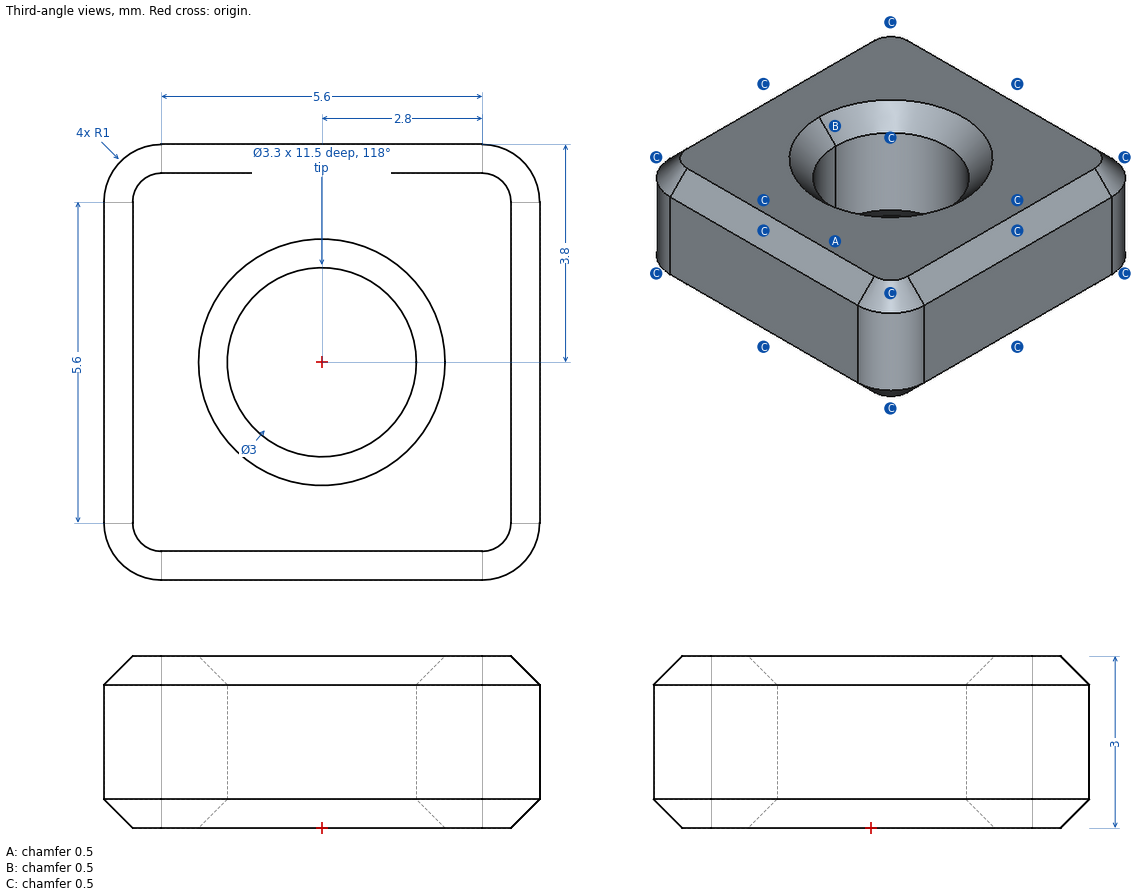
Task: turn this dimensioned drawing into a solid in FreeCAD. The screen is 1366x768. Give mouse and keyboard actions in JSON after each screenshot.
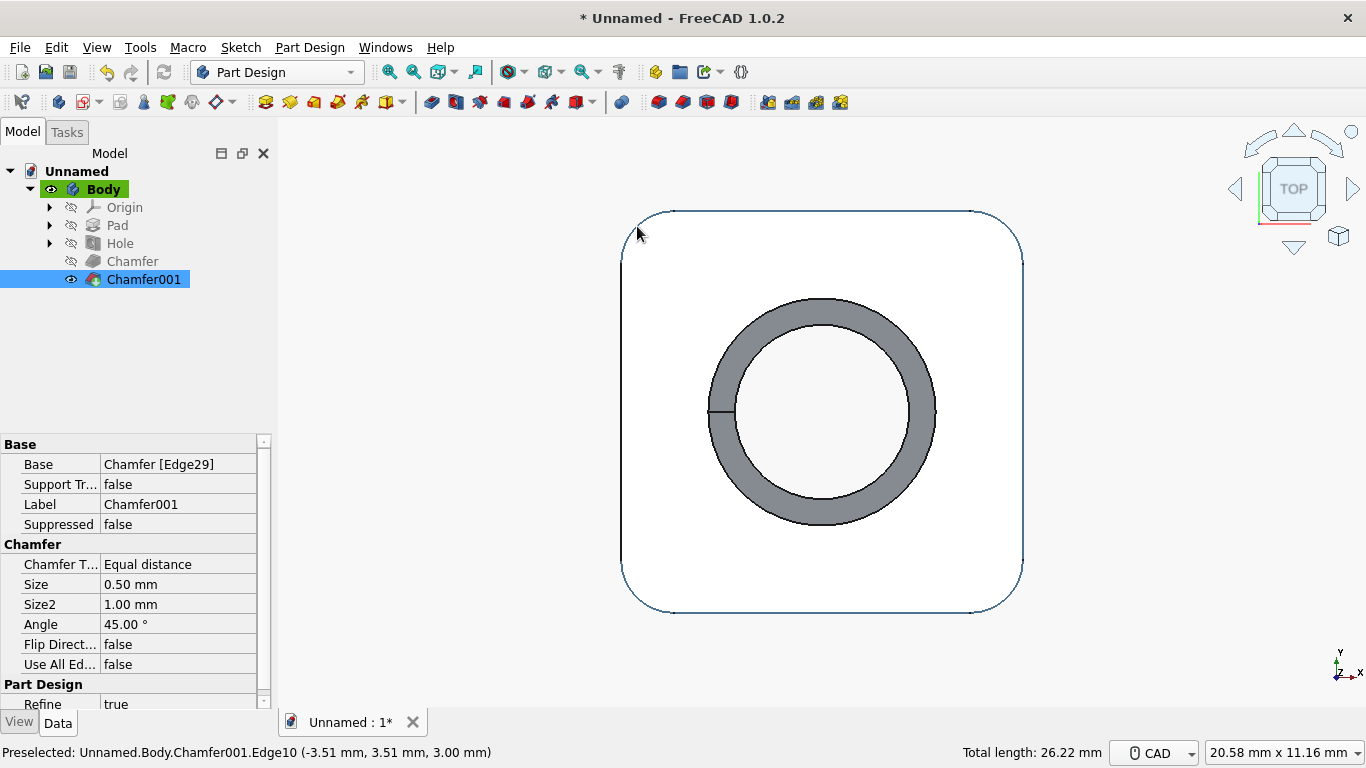
{"action": "left_click", "coordinate": [621, 411], "text": "ctrl"}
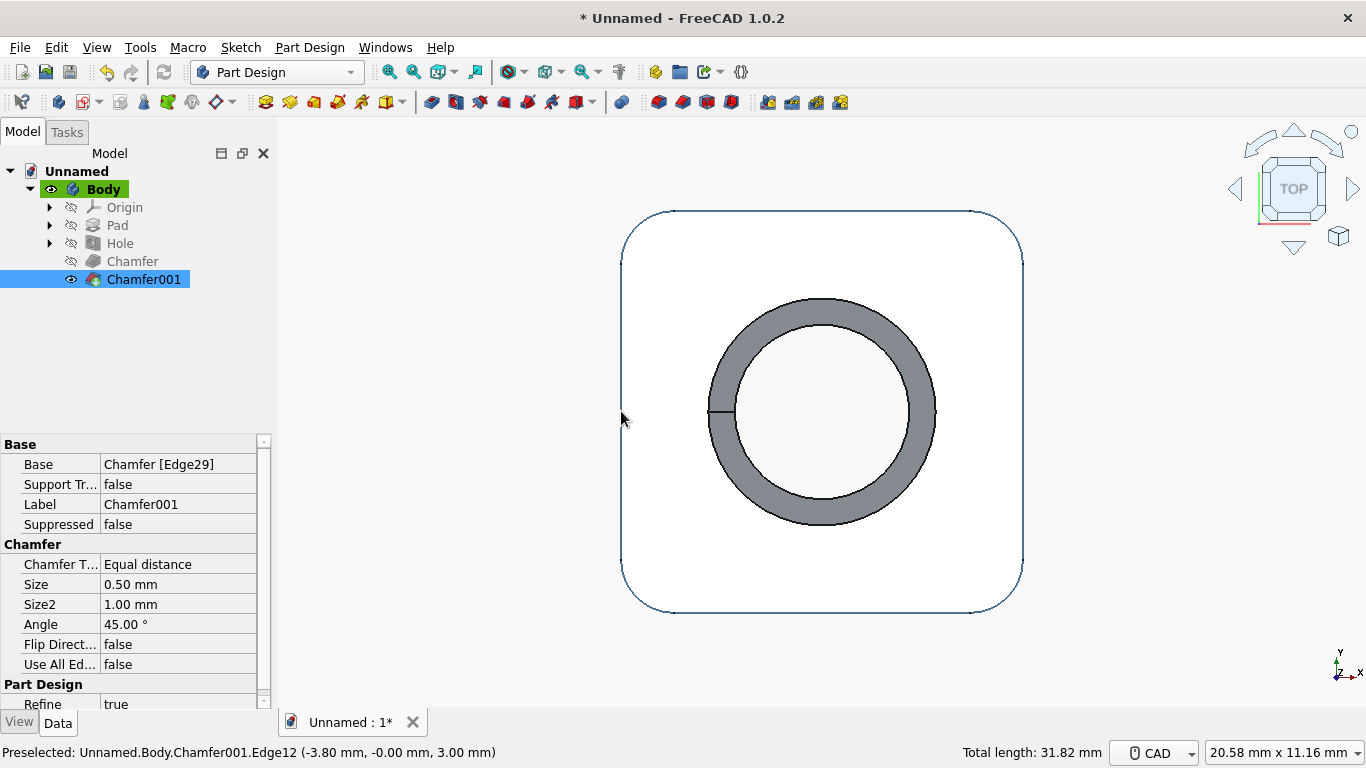
{"action": "key", "text": "0"}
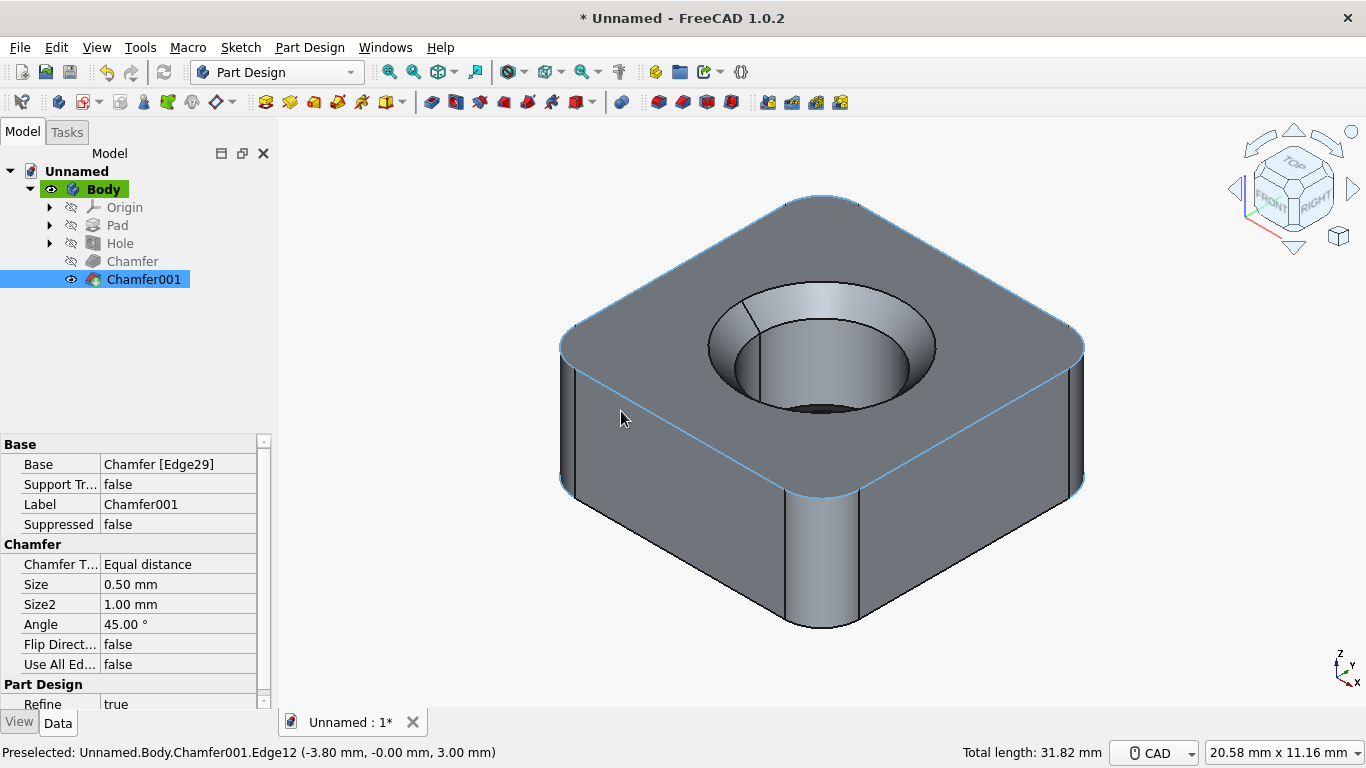
{"action": "key", "text": "1"}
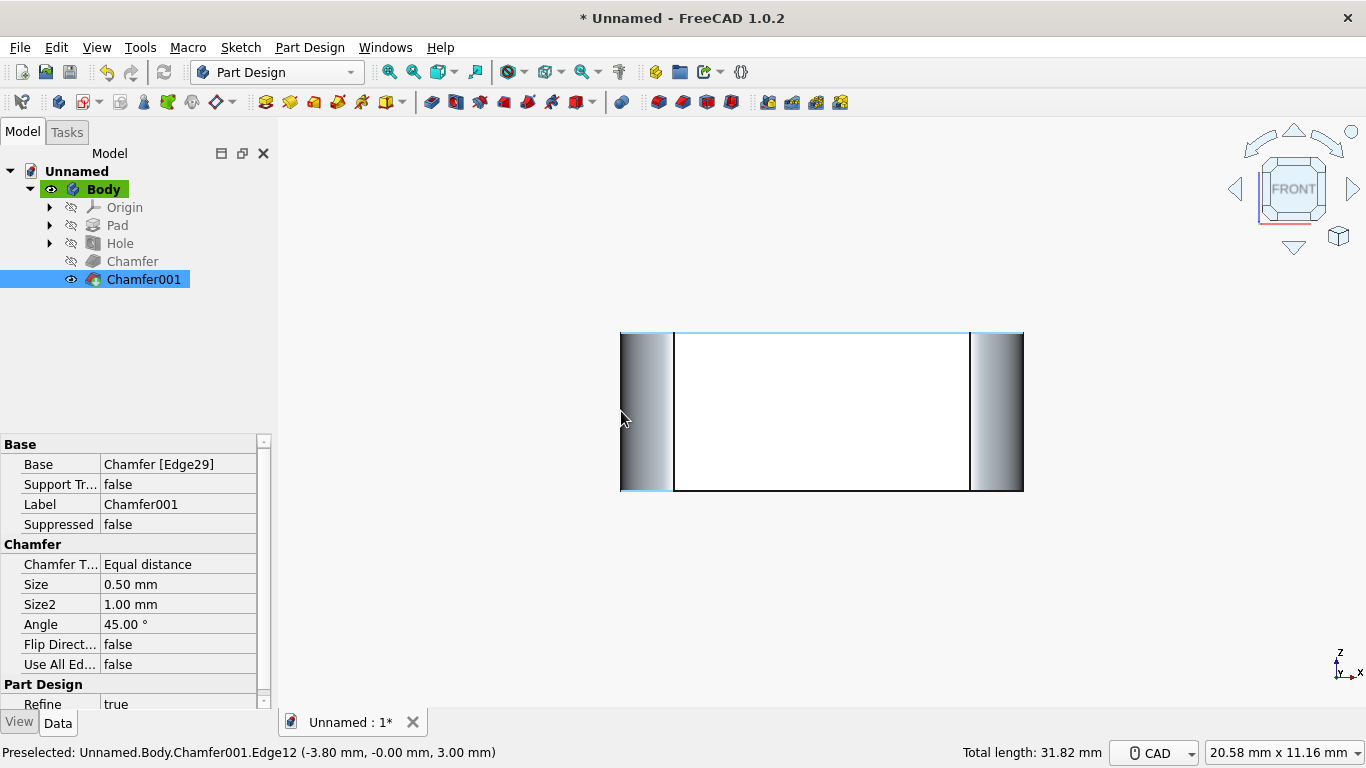
{"action": "key", "text": "v f"}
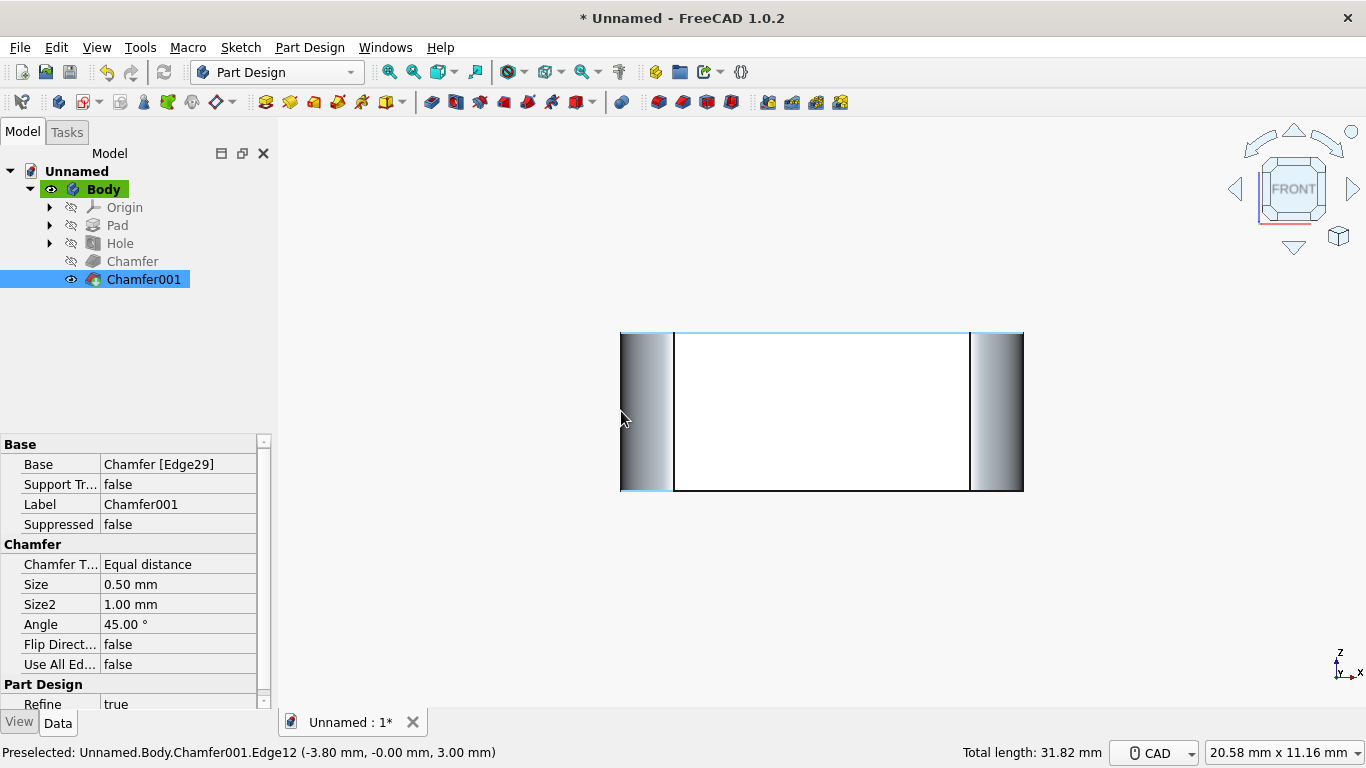
{"action": "left_click", "coordinate": [822, 490], "text": "ctrl"}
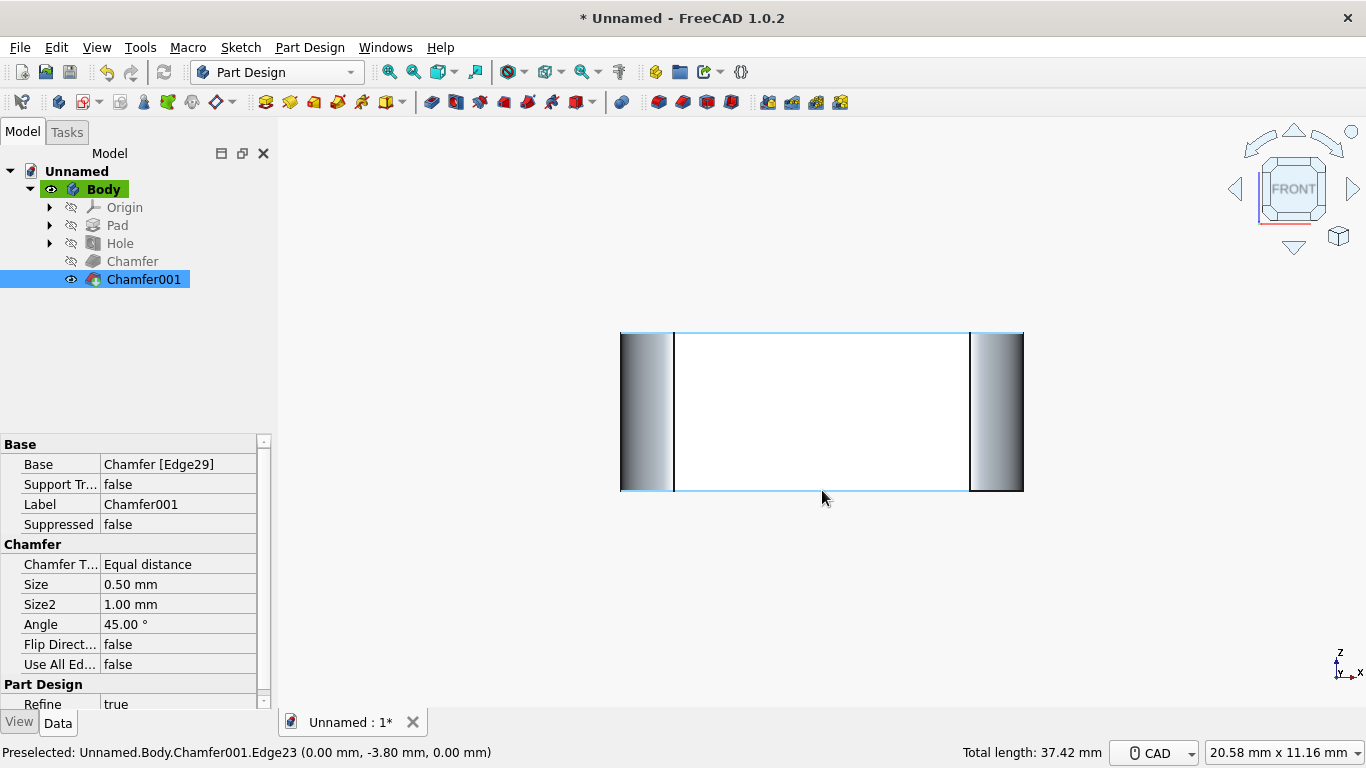
{"action": "left_click", "coordinate": [1007, 490], "text": "ctrl"}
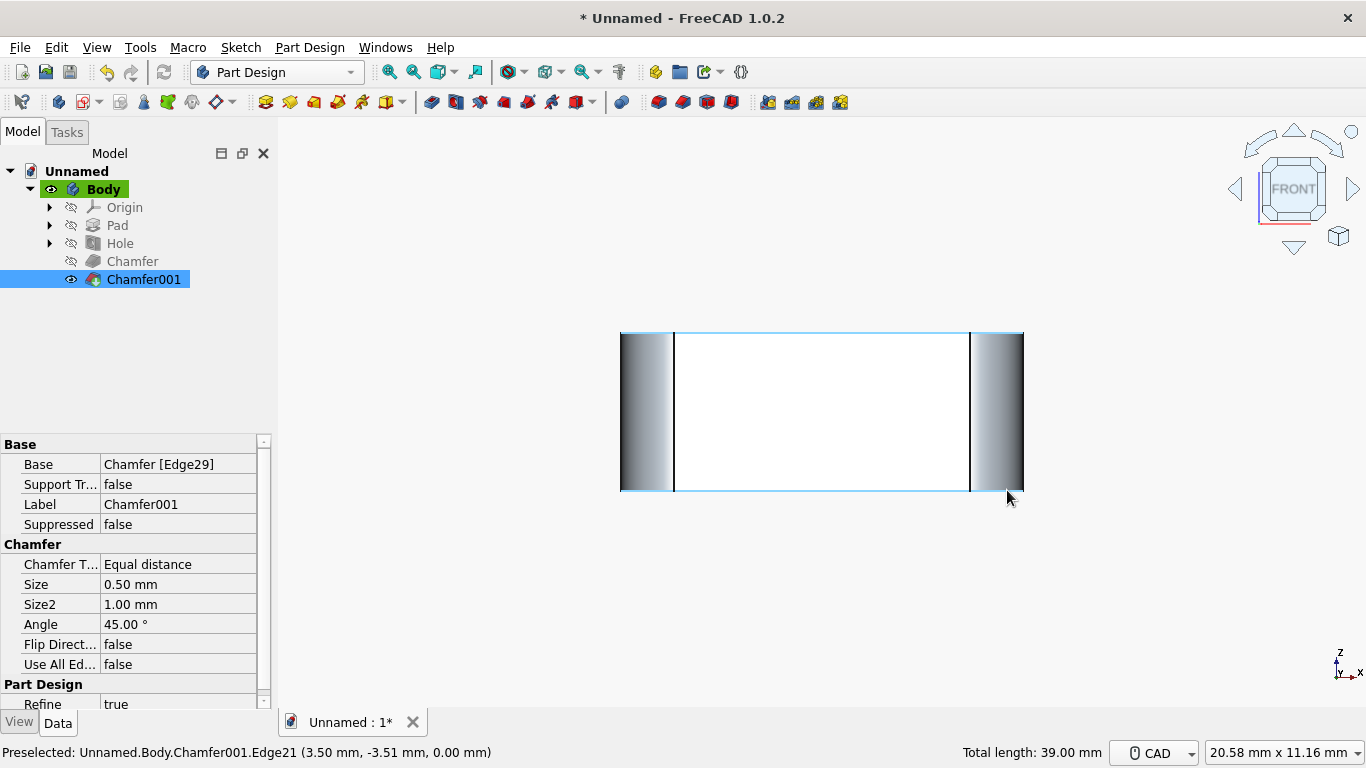
{"action": "key", "text": "3"}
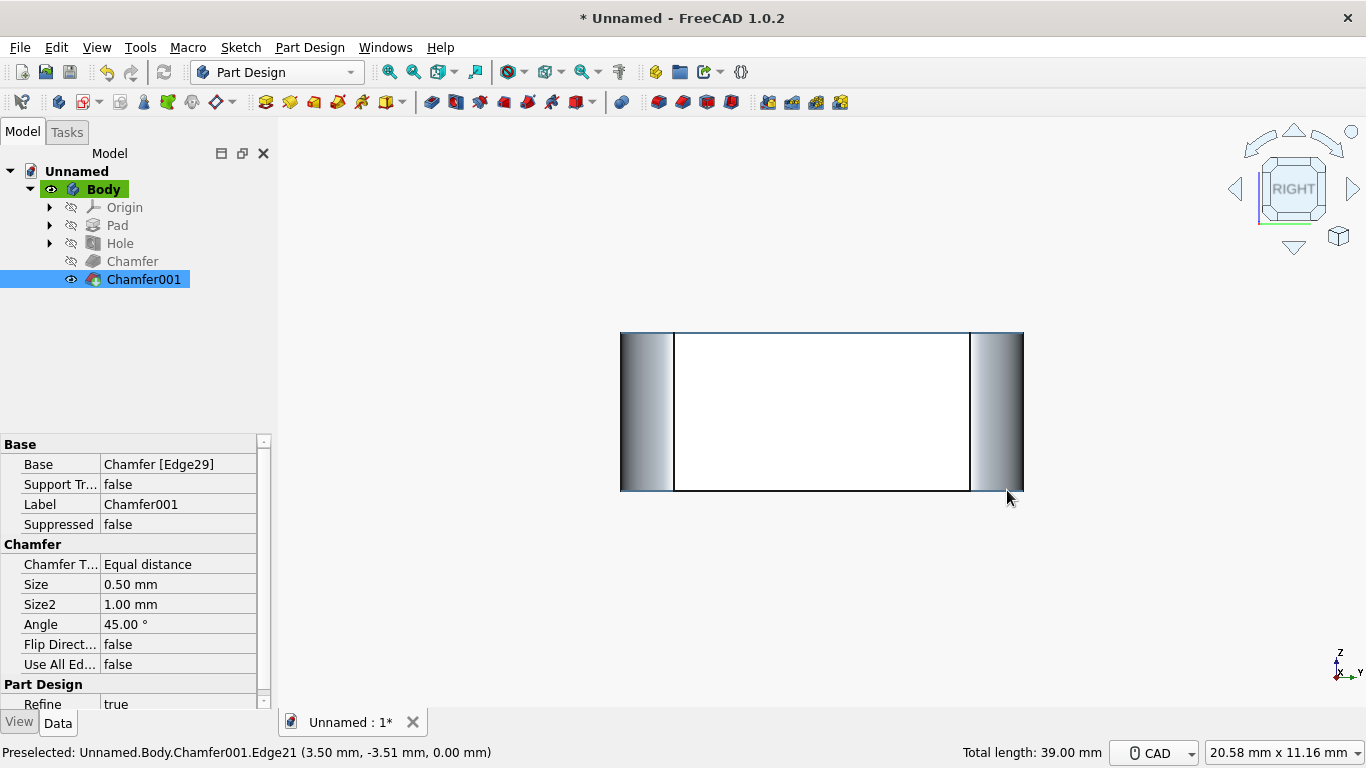
{"action": "left_click", "coordinate": [390, 72]}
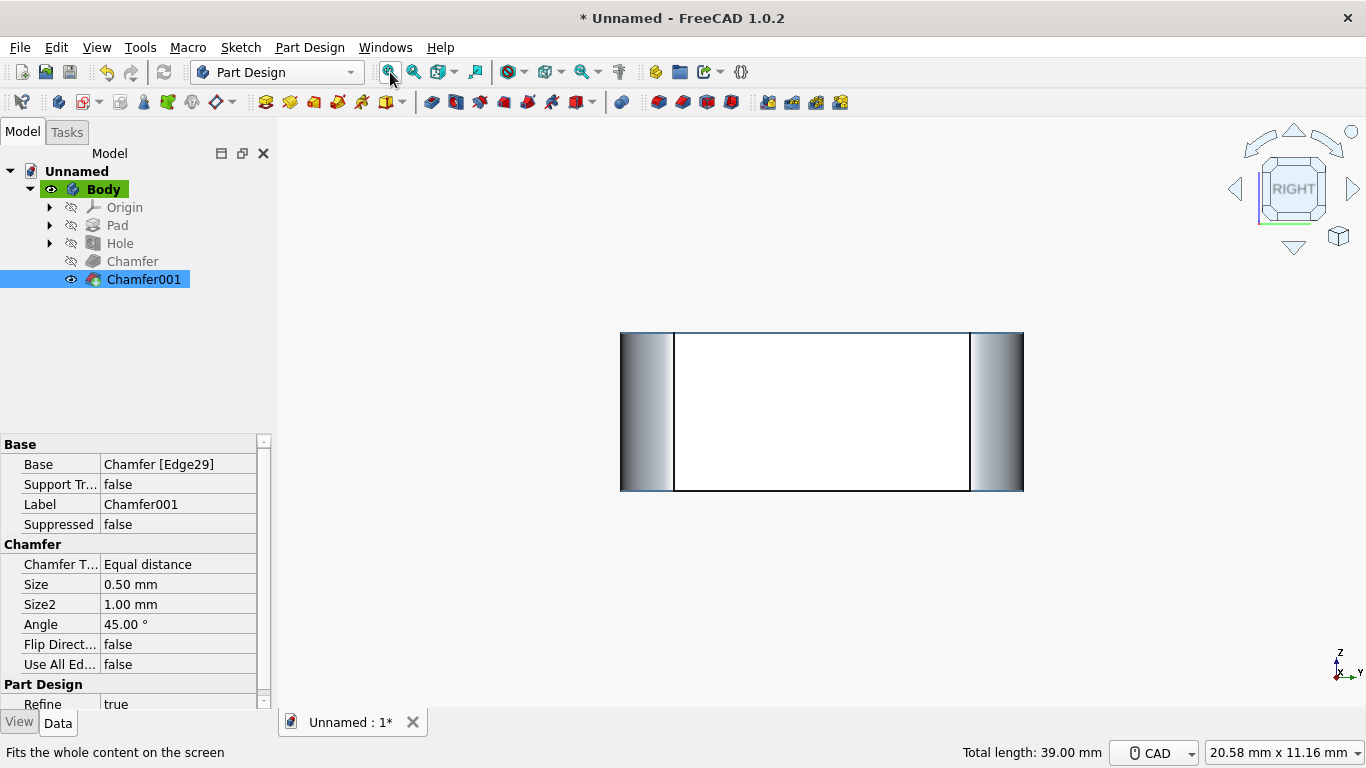
{"action": "left_click", "coordinate": [822, 490], "text": "ctrl"}